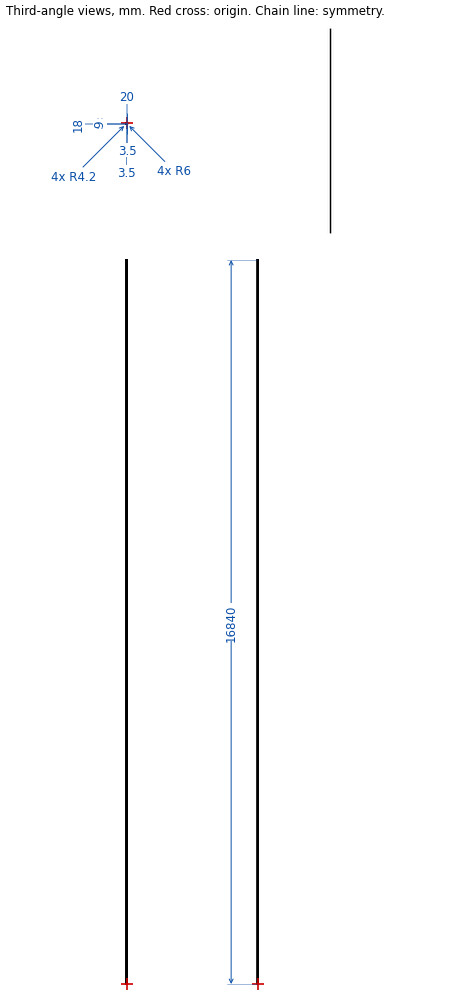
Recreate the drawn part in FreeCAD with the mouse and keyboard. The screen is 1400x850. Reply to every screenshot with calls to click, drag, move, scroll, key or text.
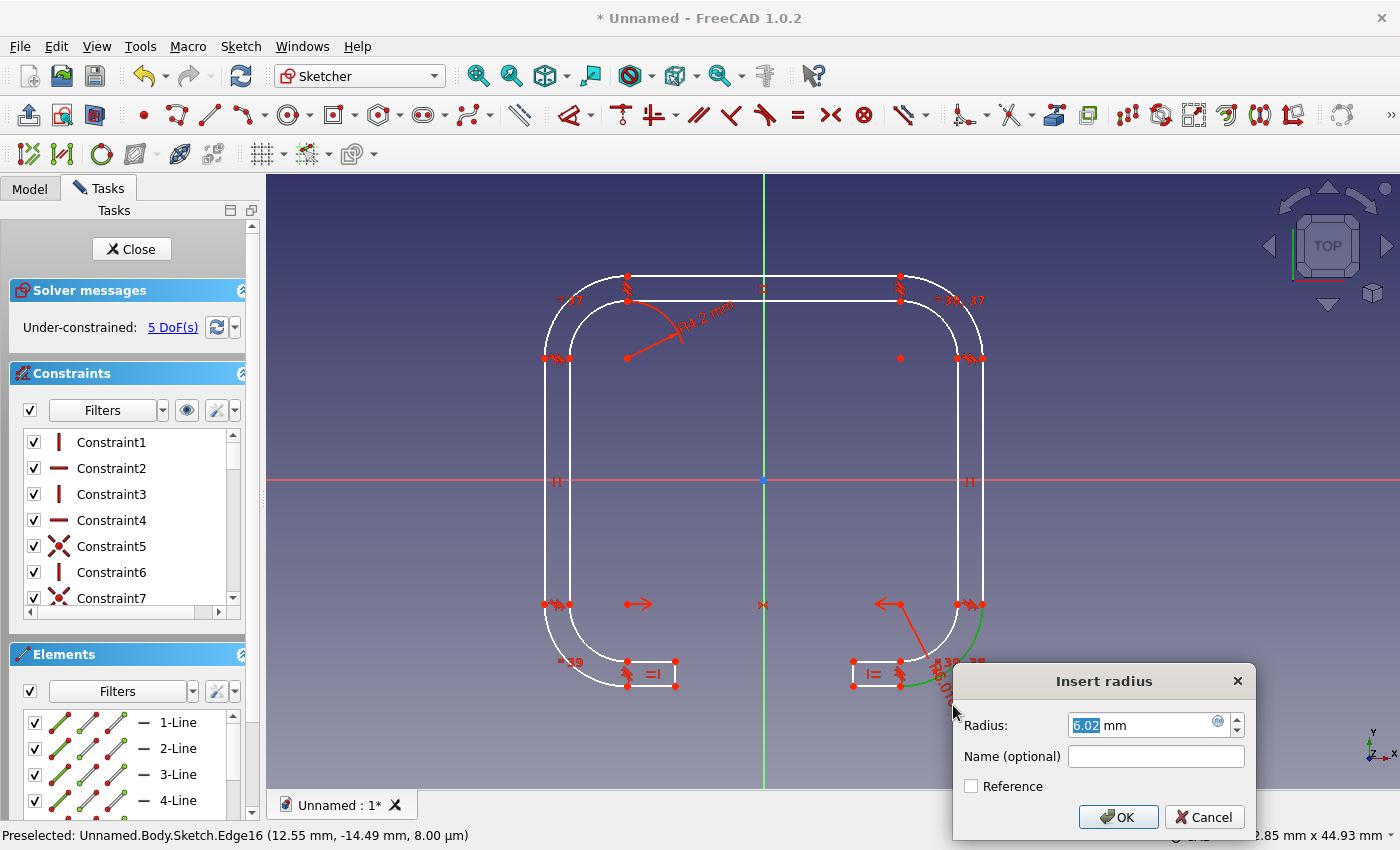
text(6)
key(Return)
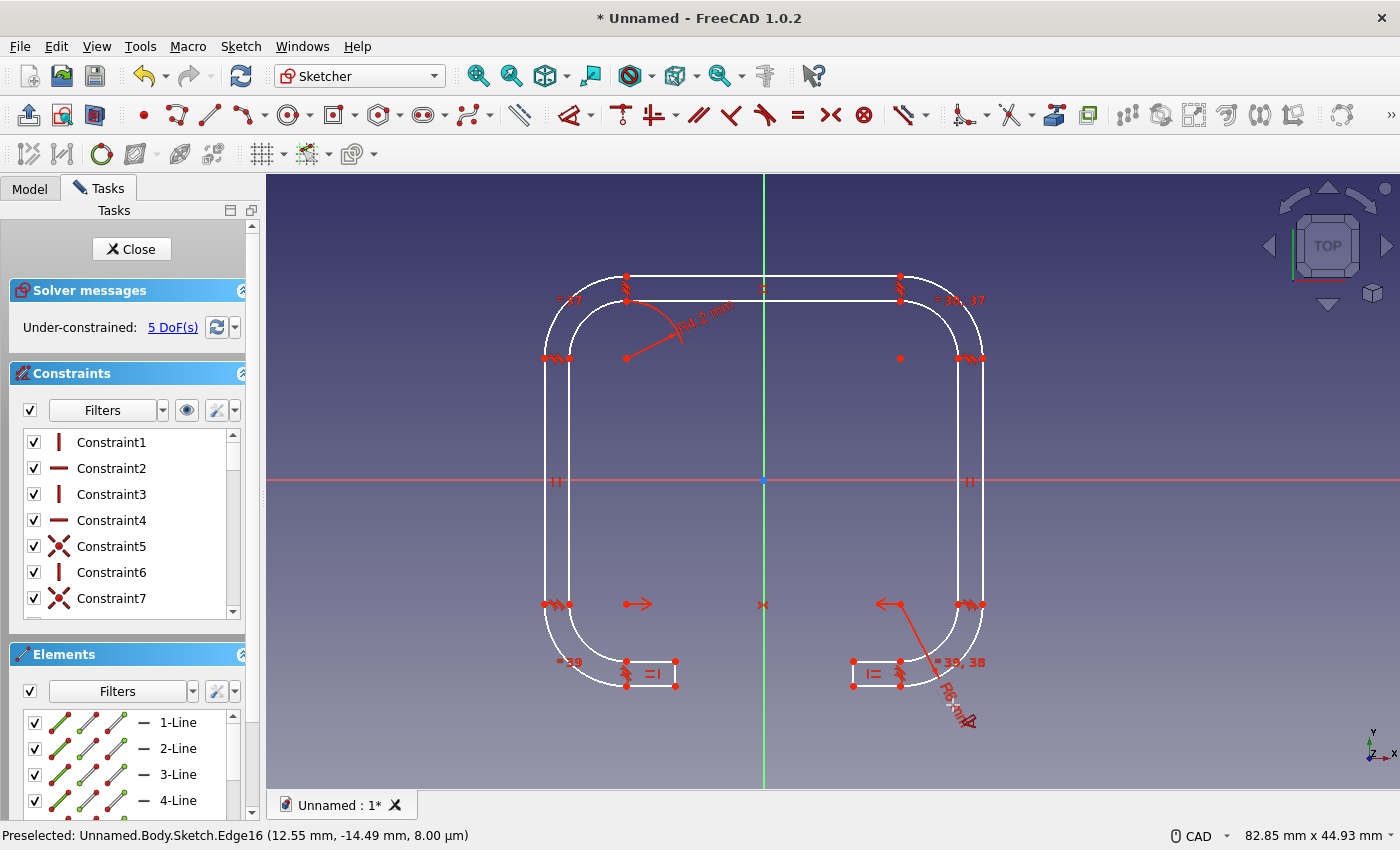
click(569, 530)
click(603, 425)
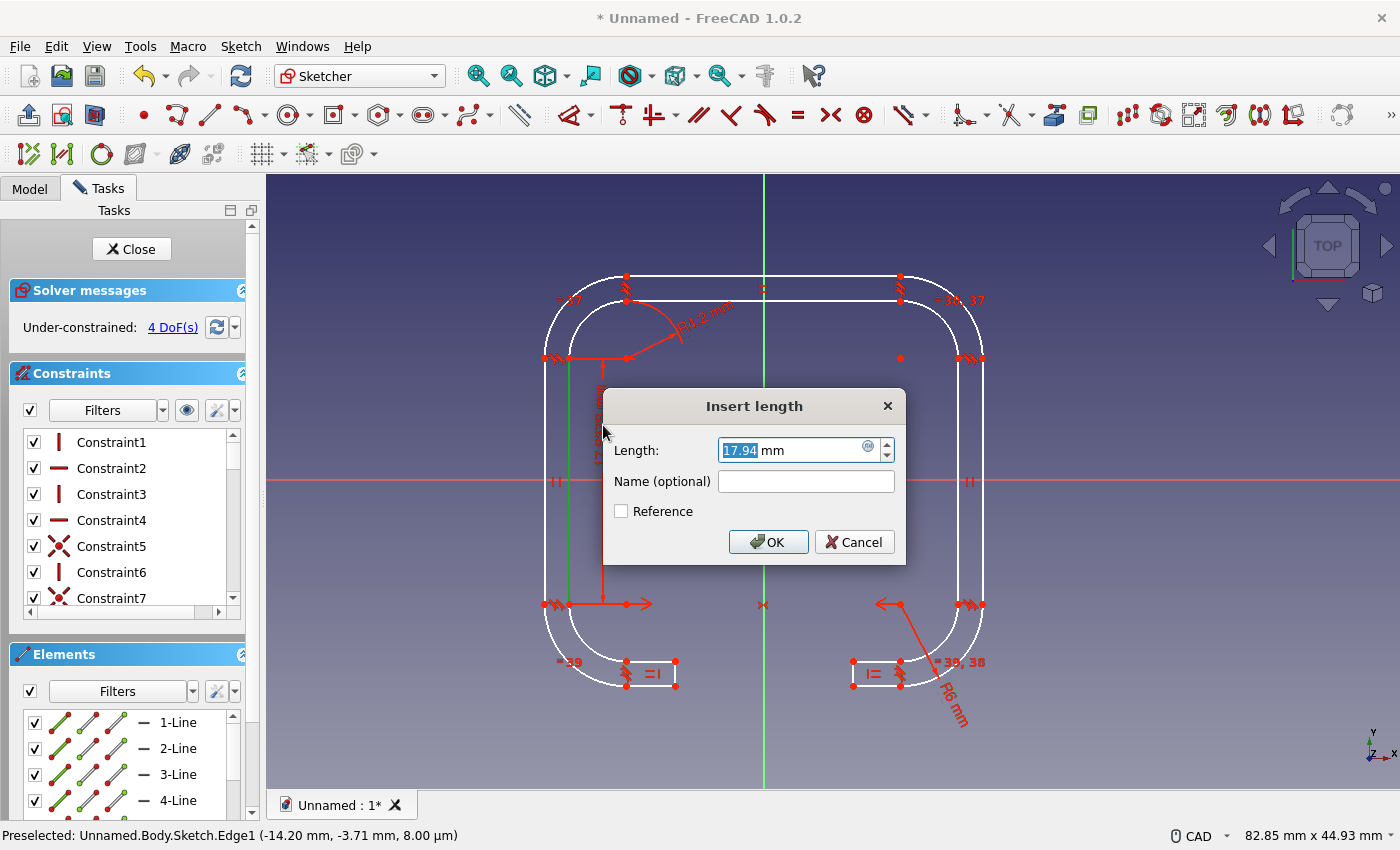
text(18)
key(Return)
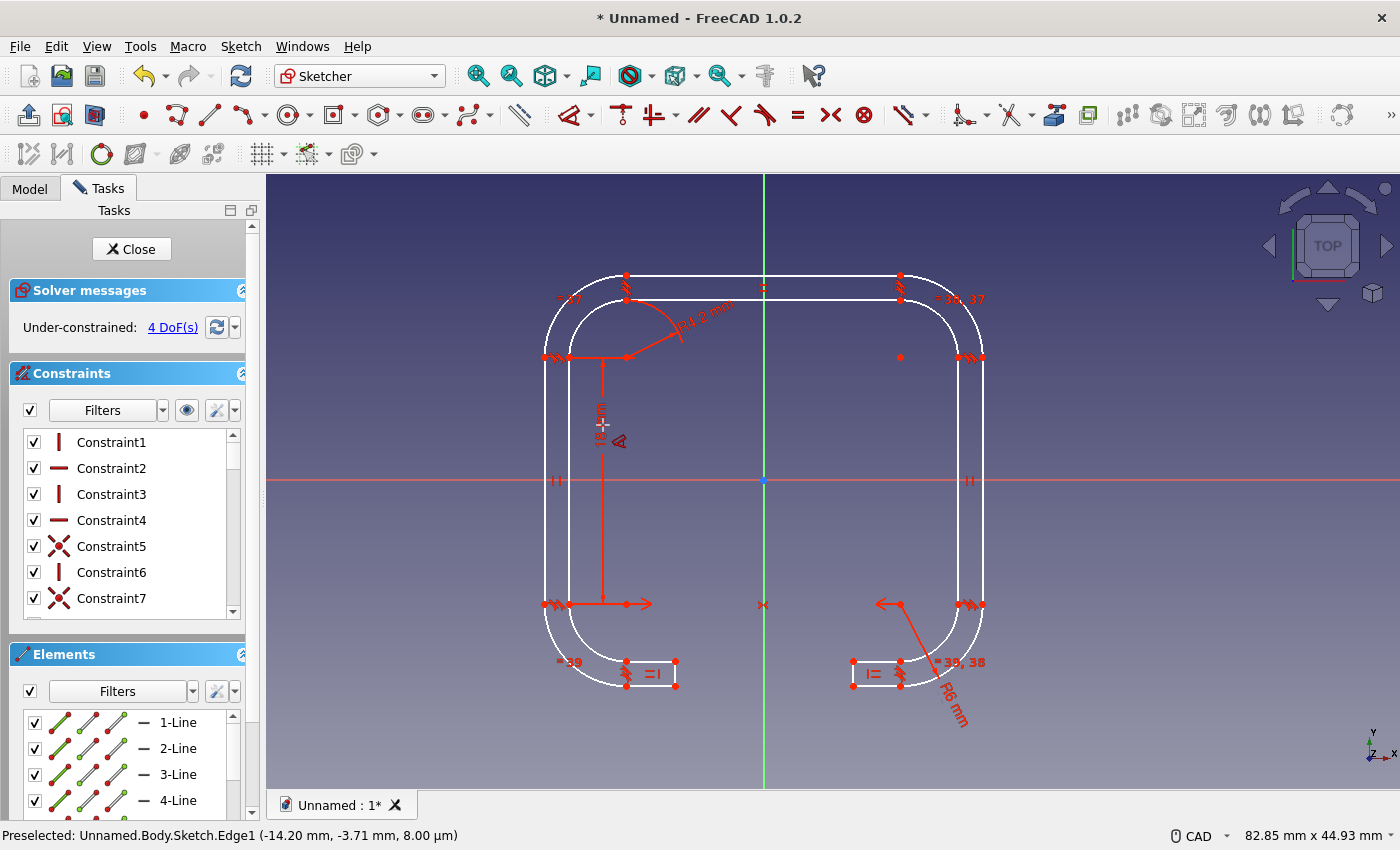
click(709, 300)
click(827, 334)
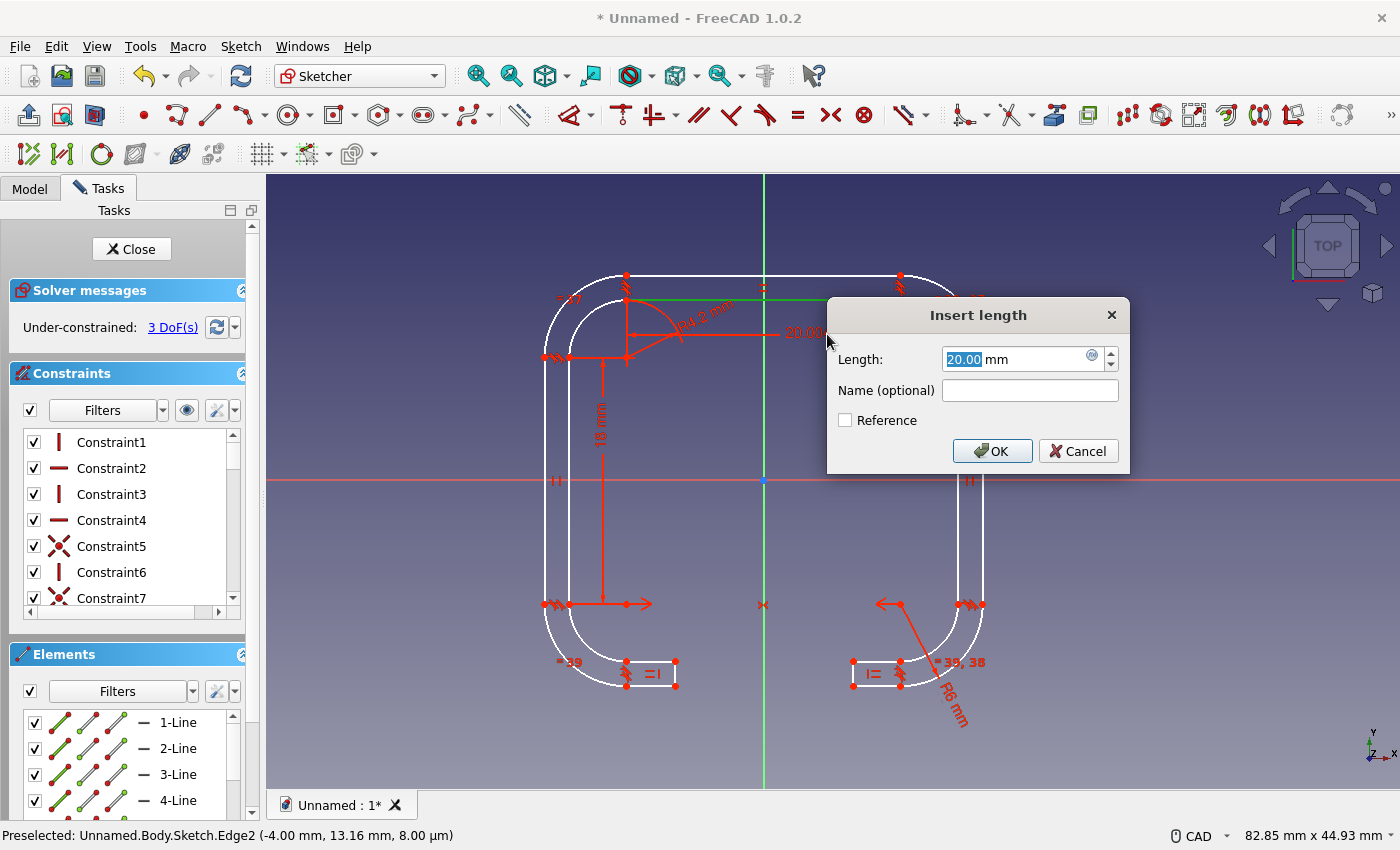
text(20)
key(Return)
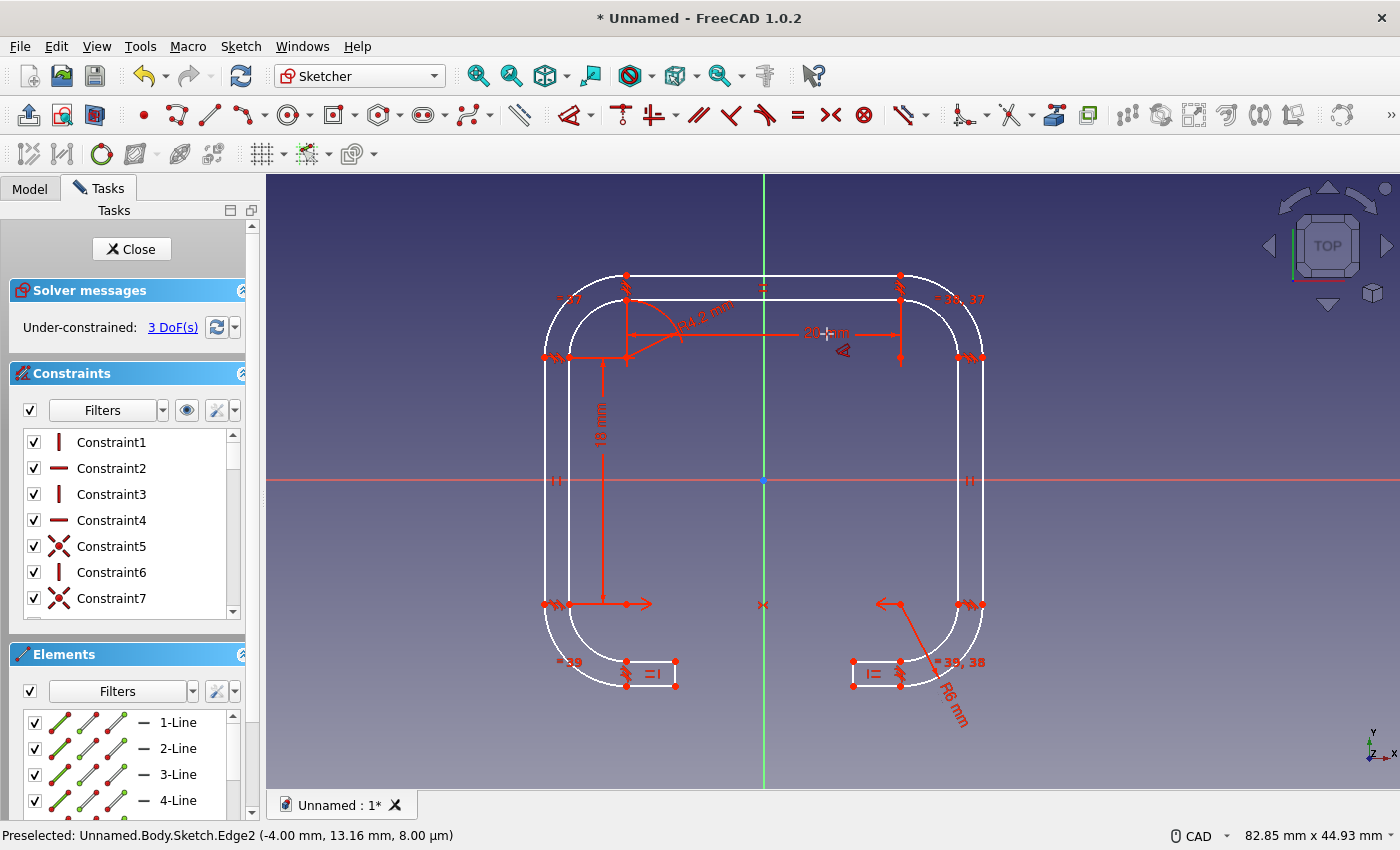
click(569, 604)
click(798, 542)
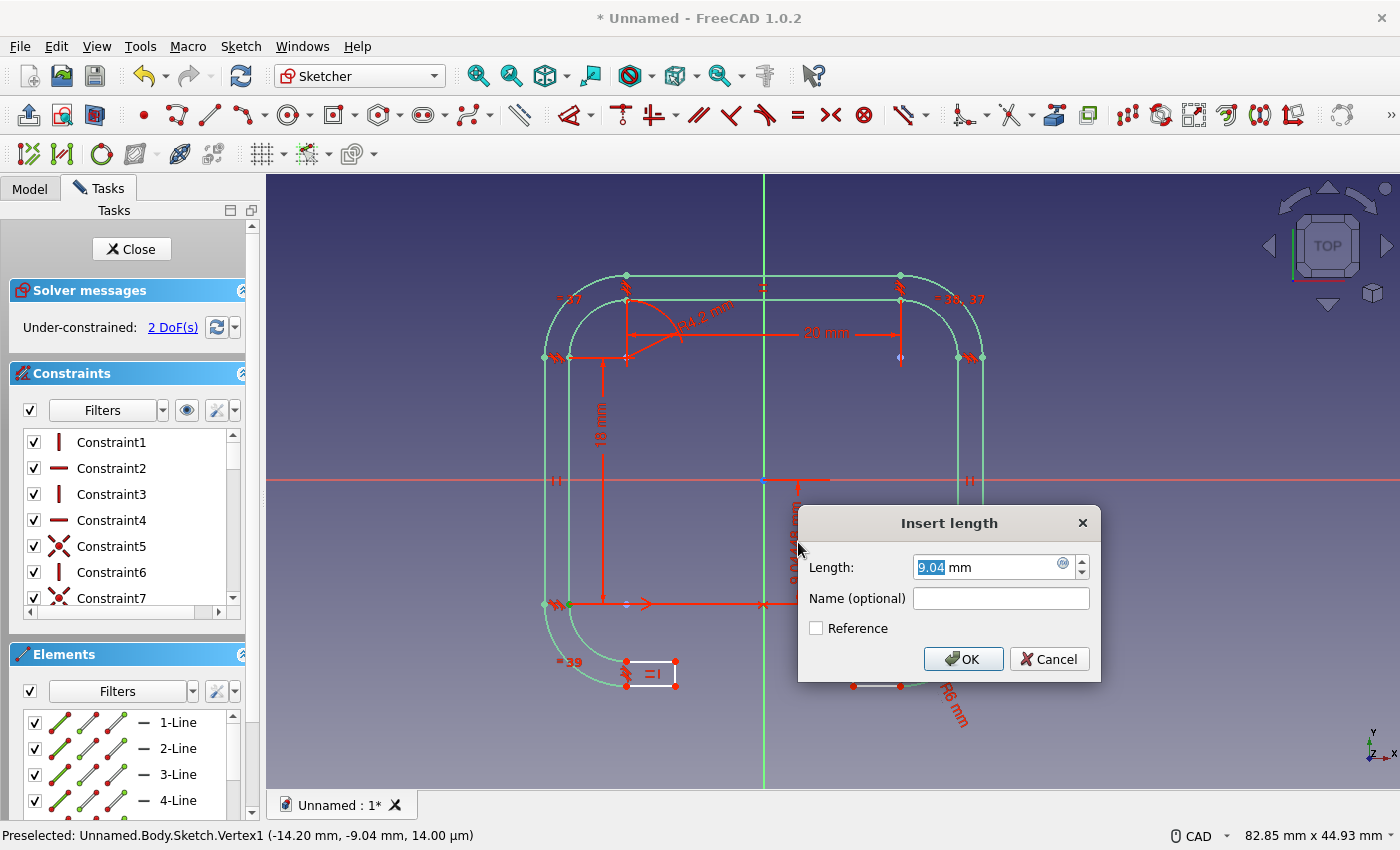
text(9)
key(Return)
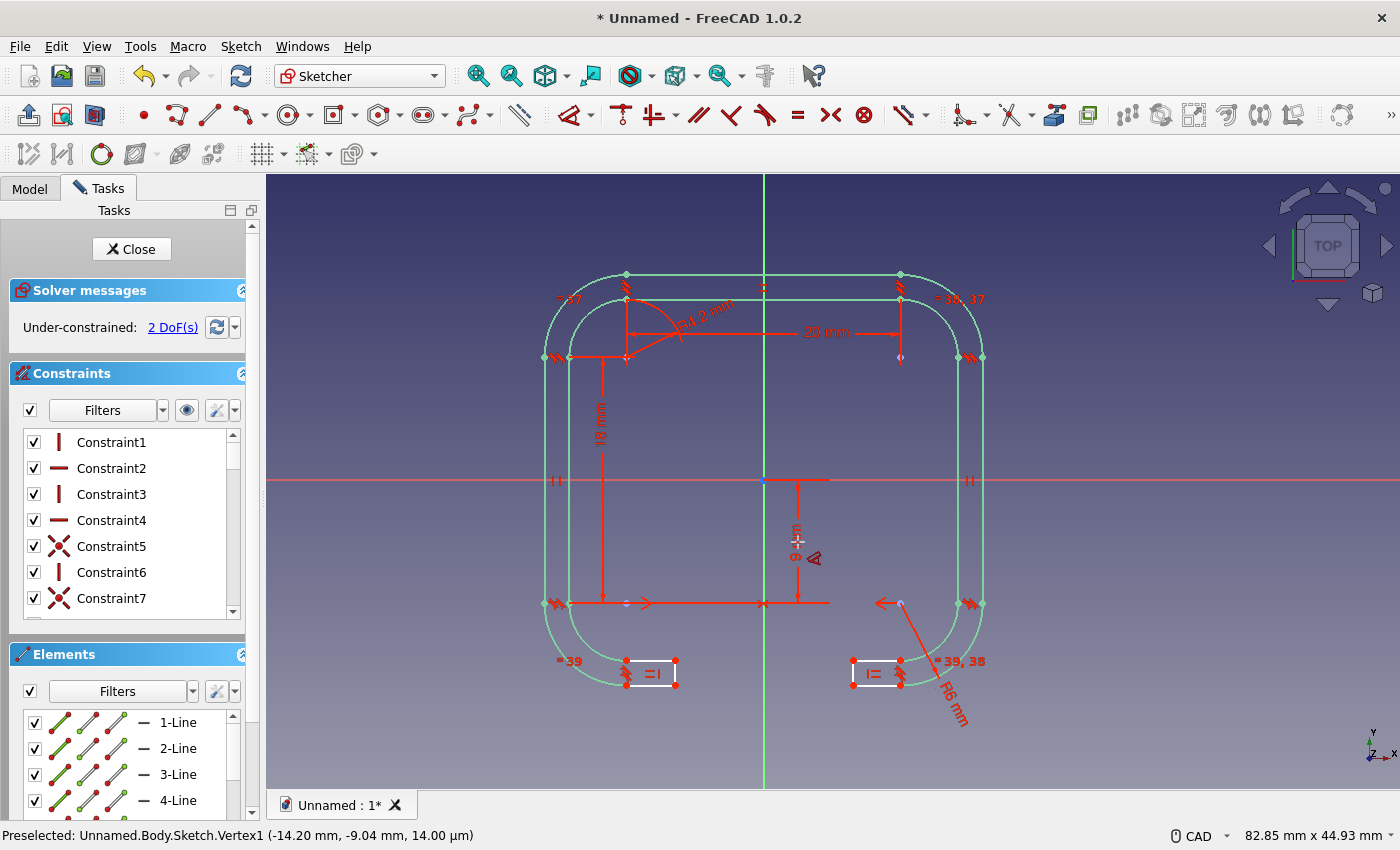
click(886, 661)
click(877, 627)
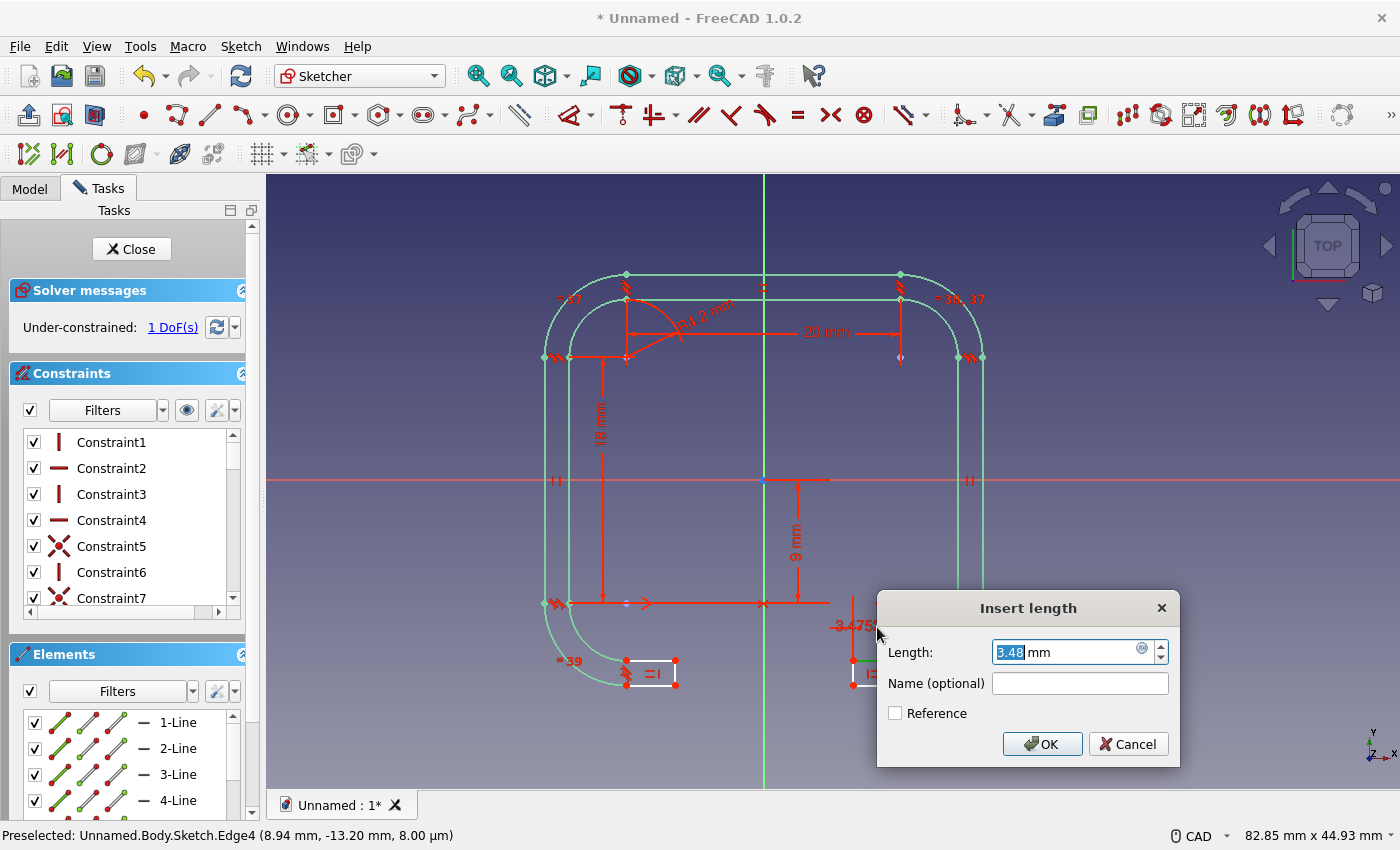
text(3.5)
key(Return)